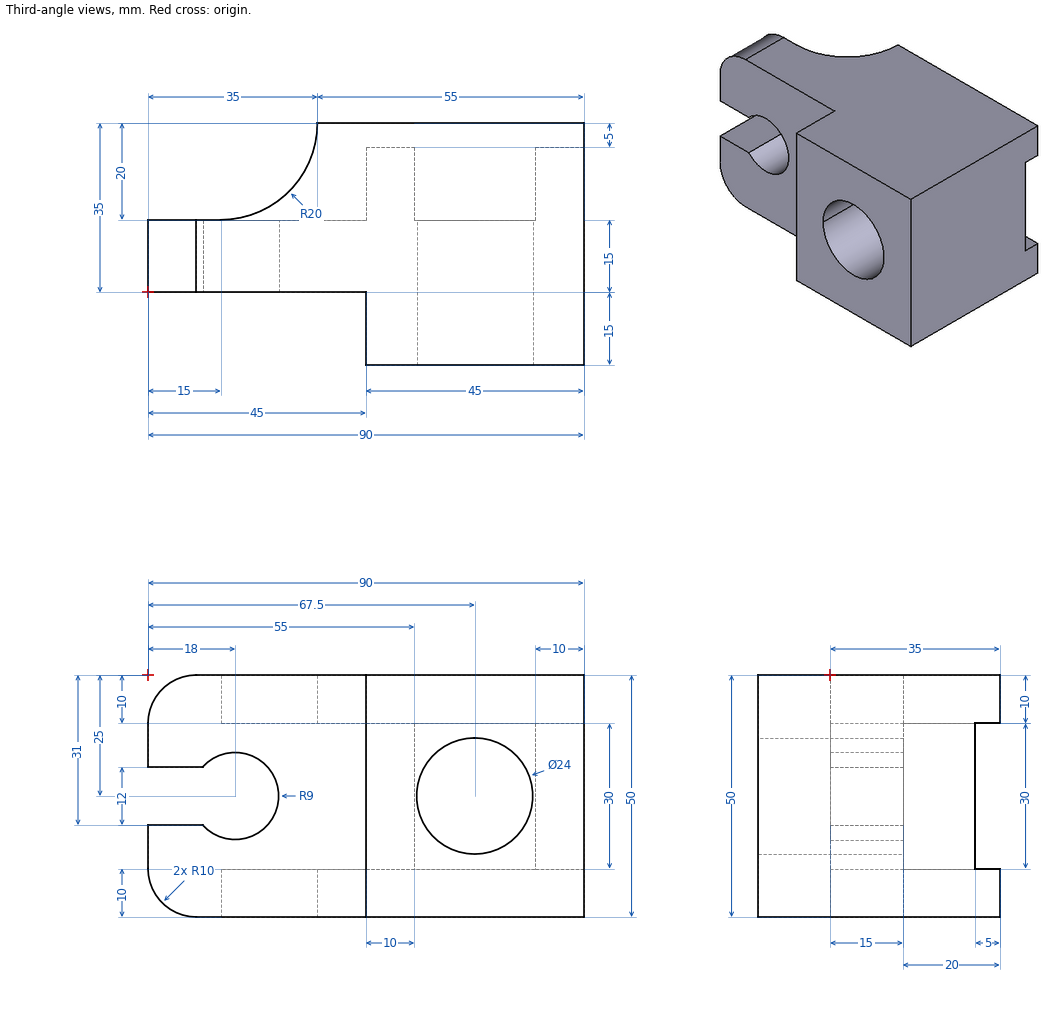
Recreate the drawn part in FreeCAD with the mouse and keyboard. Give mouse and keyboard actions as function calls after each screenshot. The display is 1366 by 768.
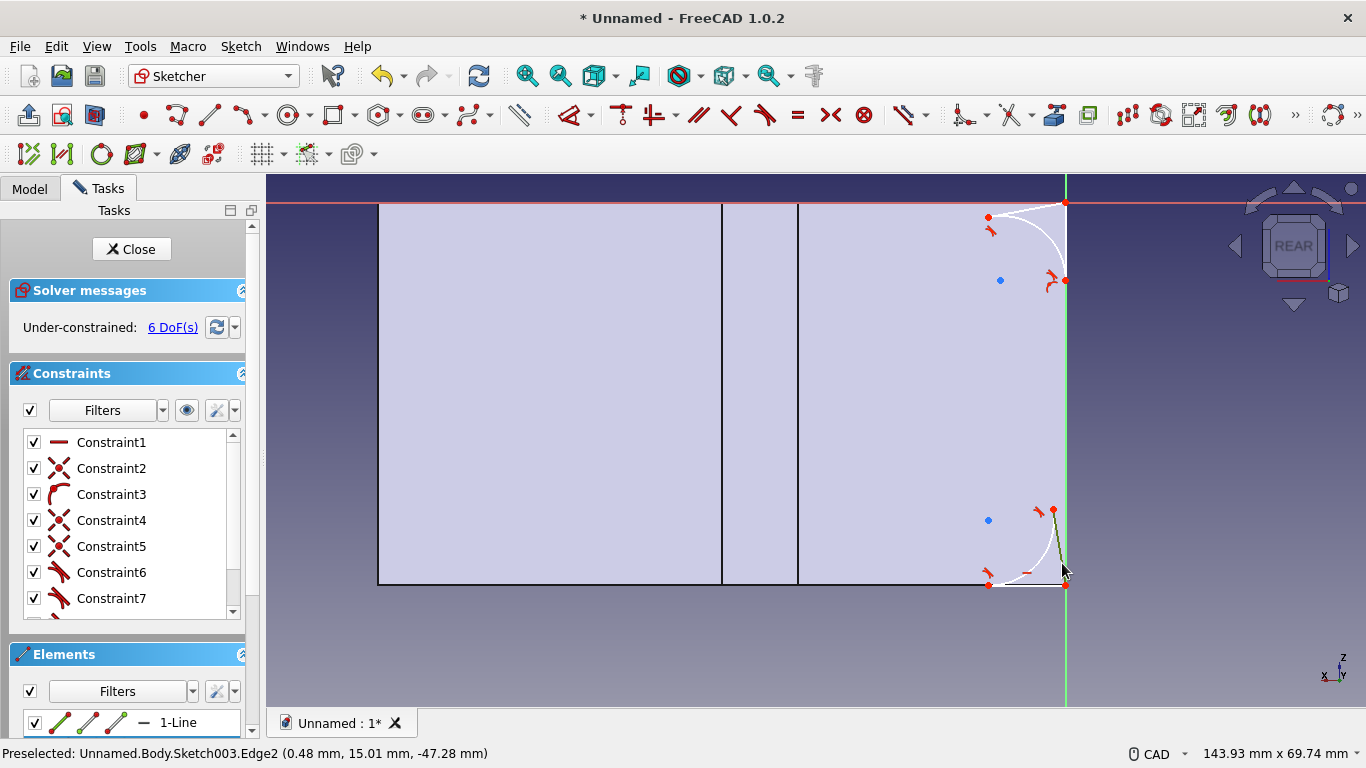
key(v)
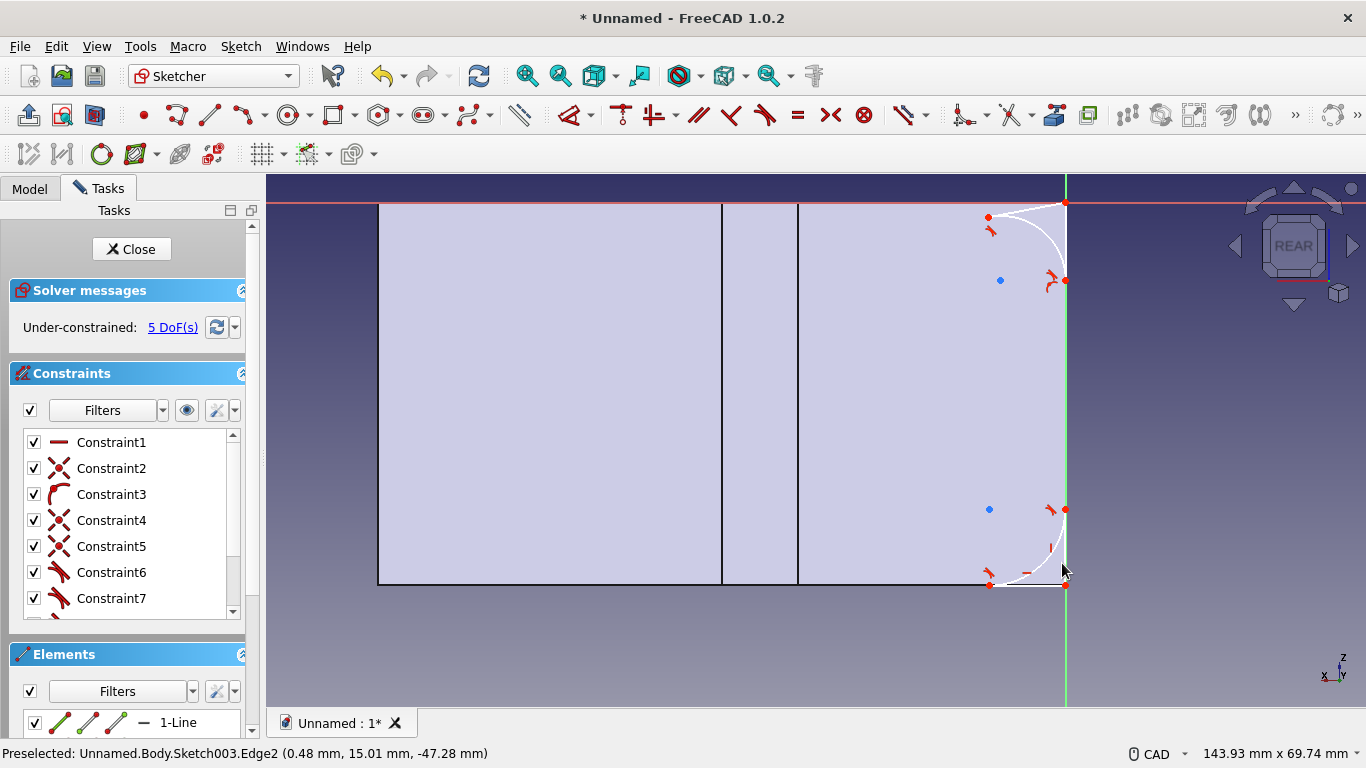
click(1050, 206)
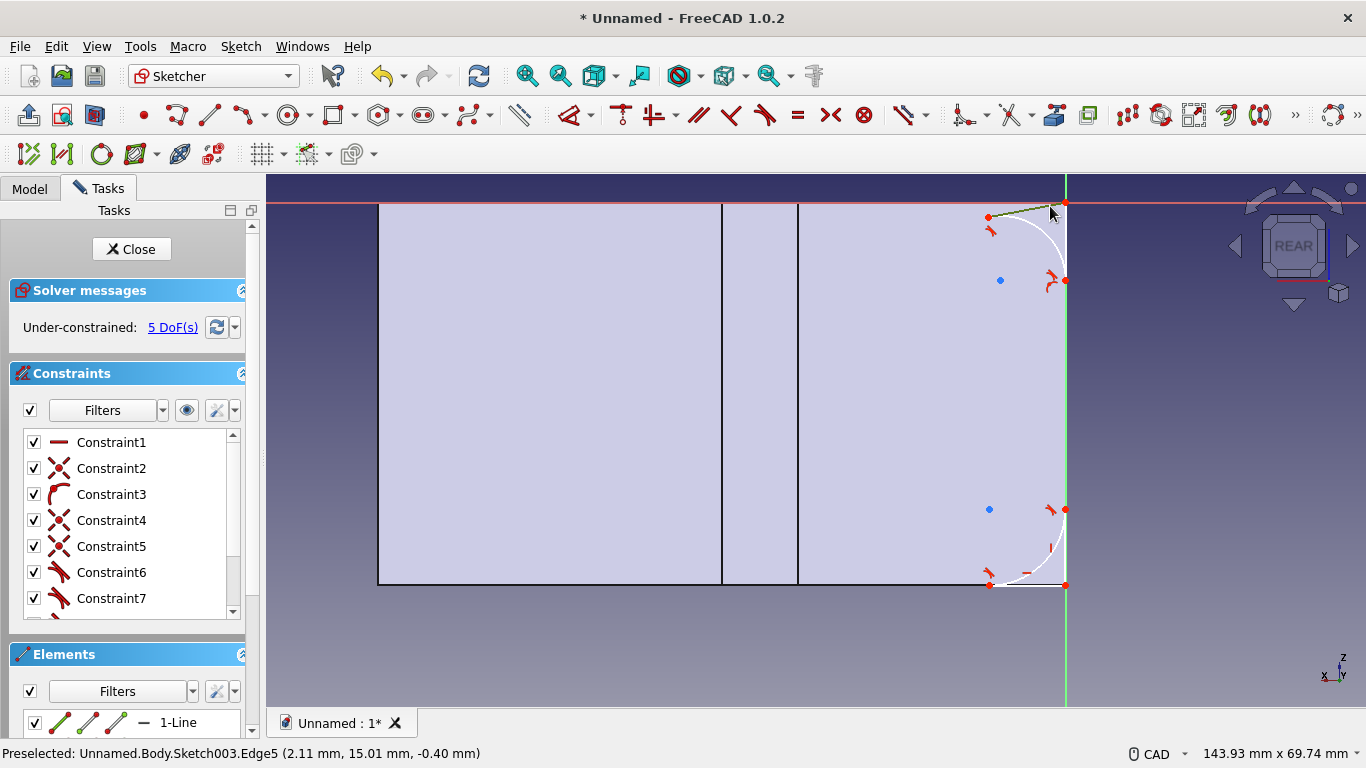
click(676, 116)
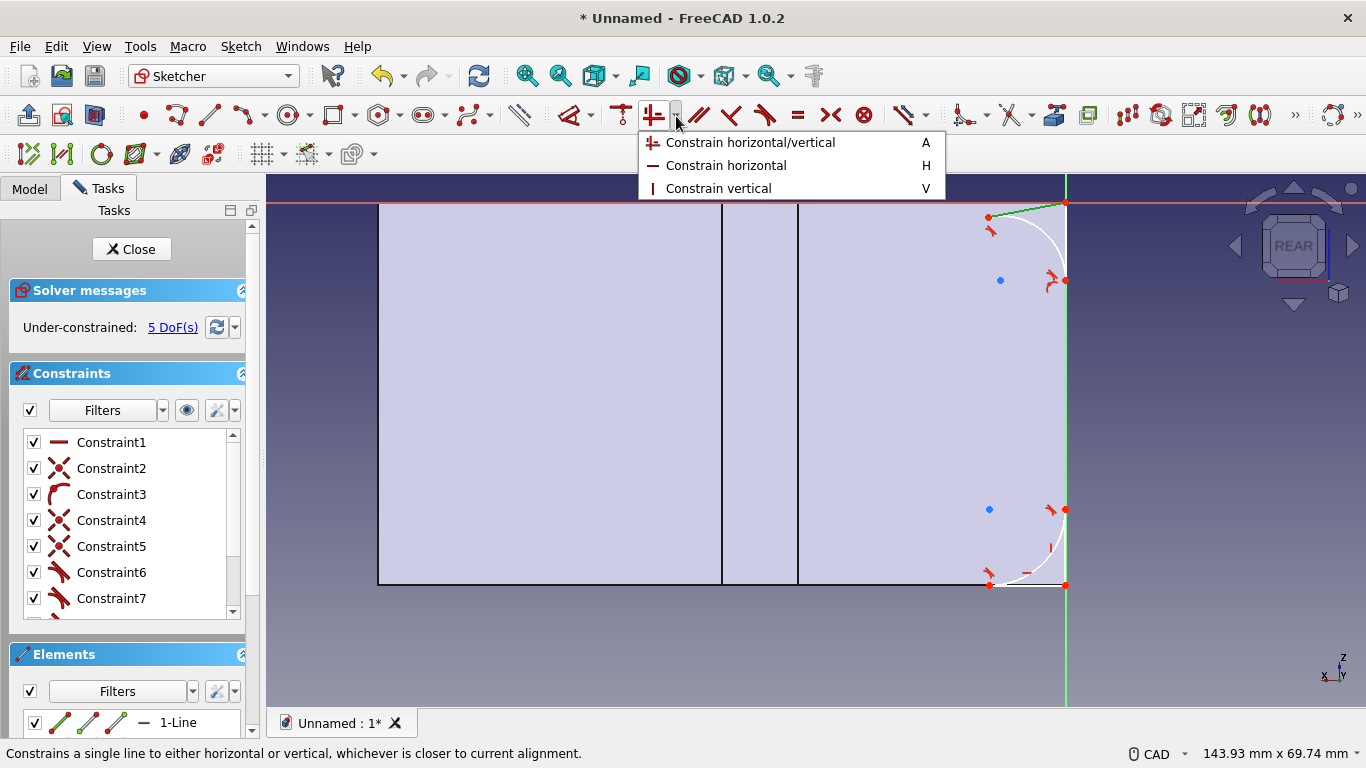
click(792, 166)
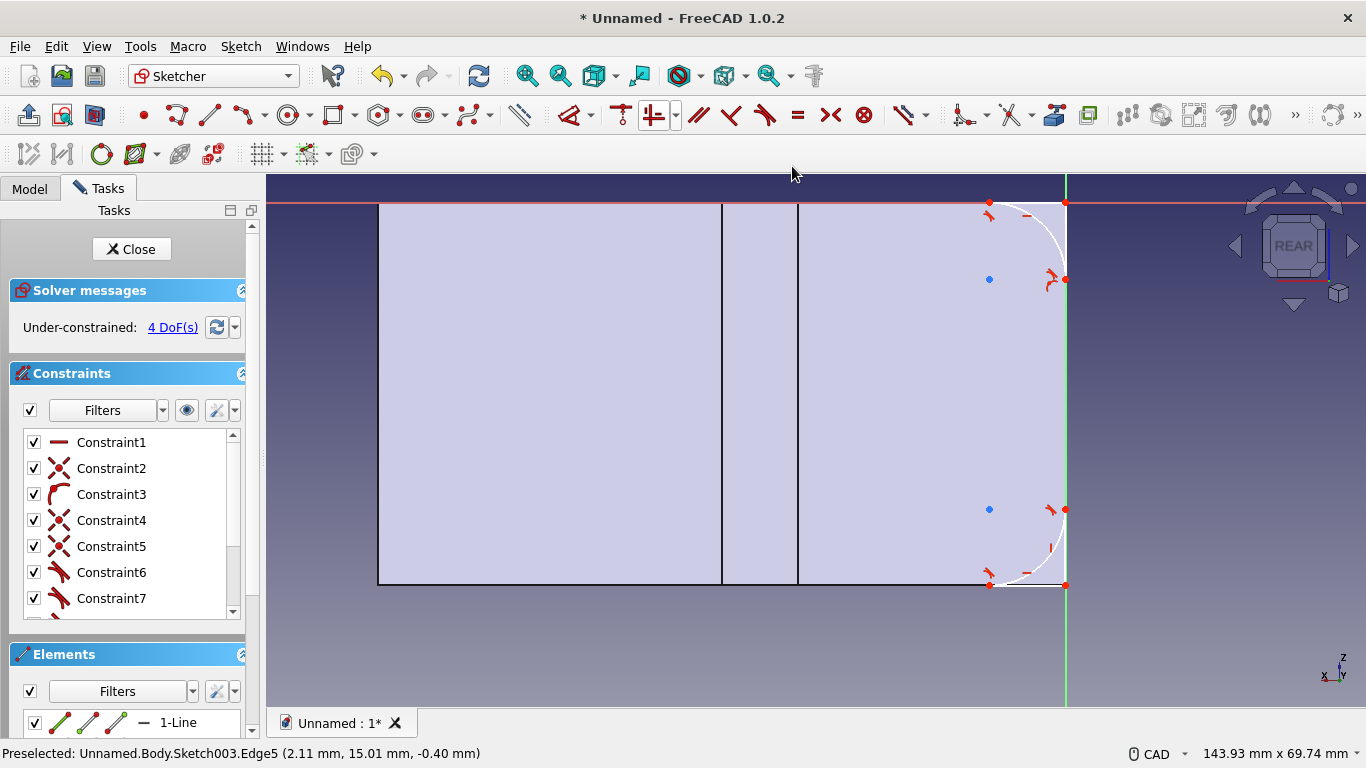
click(1043, 563)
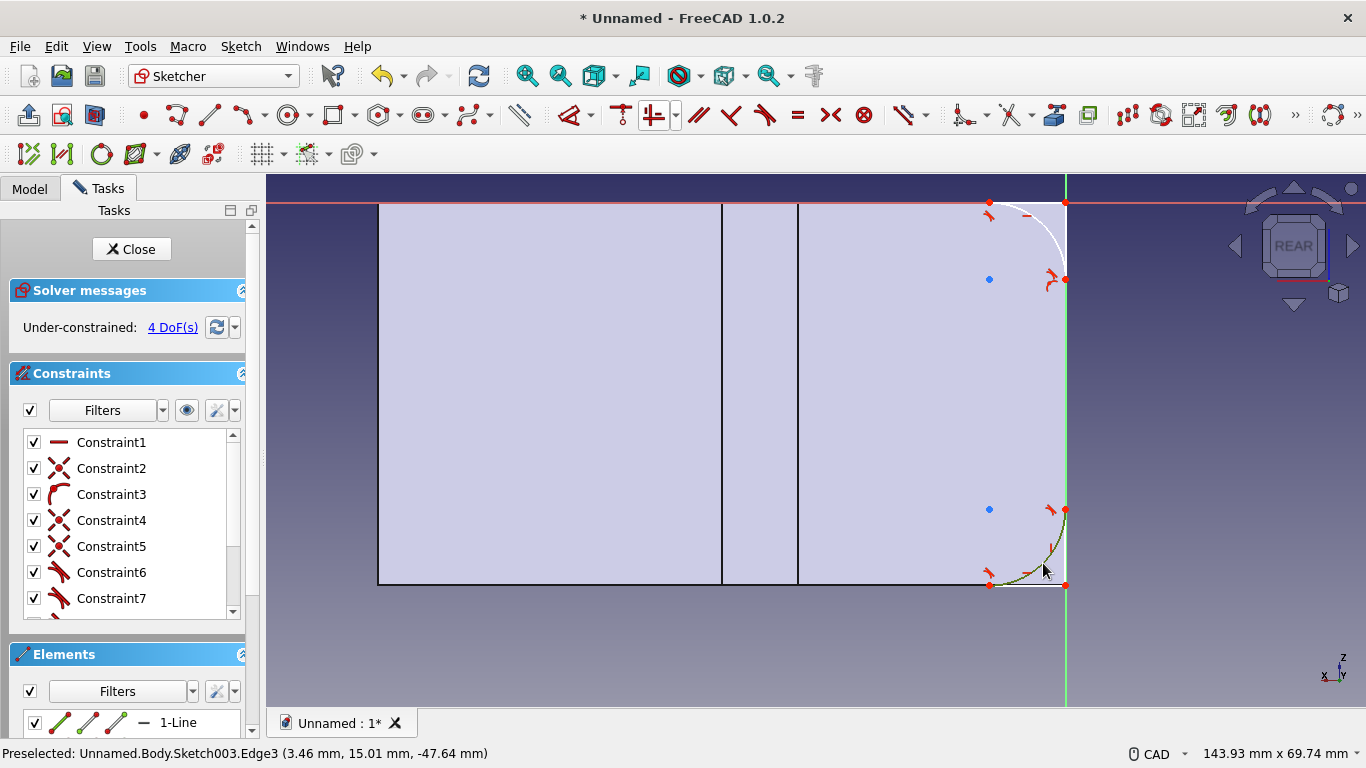
click(1043, 225)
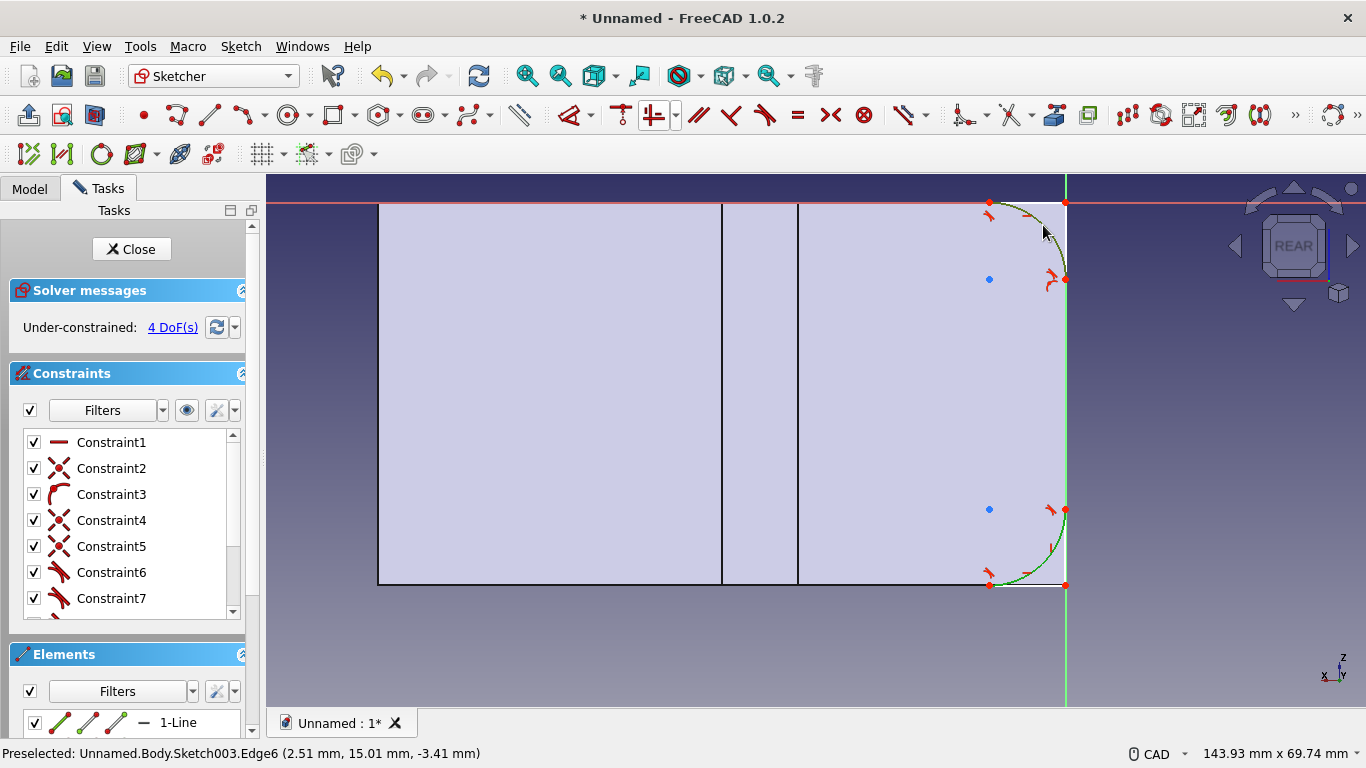
click(798, 116)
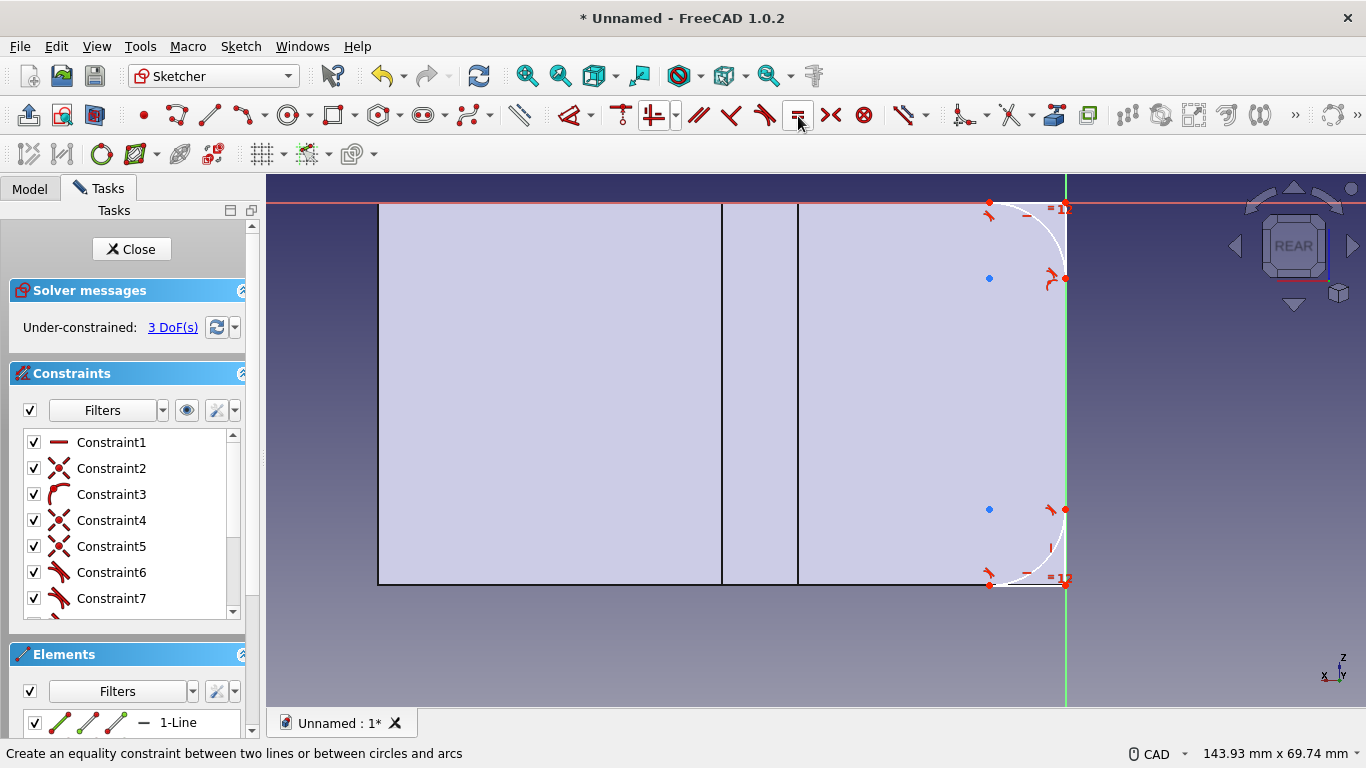
key(d)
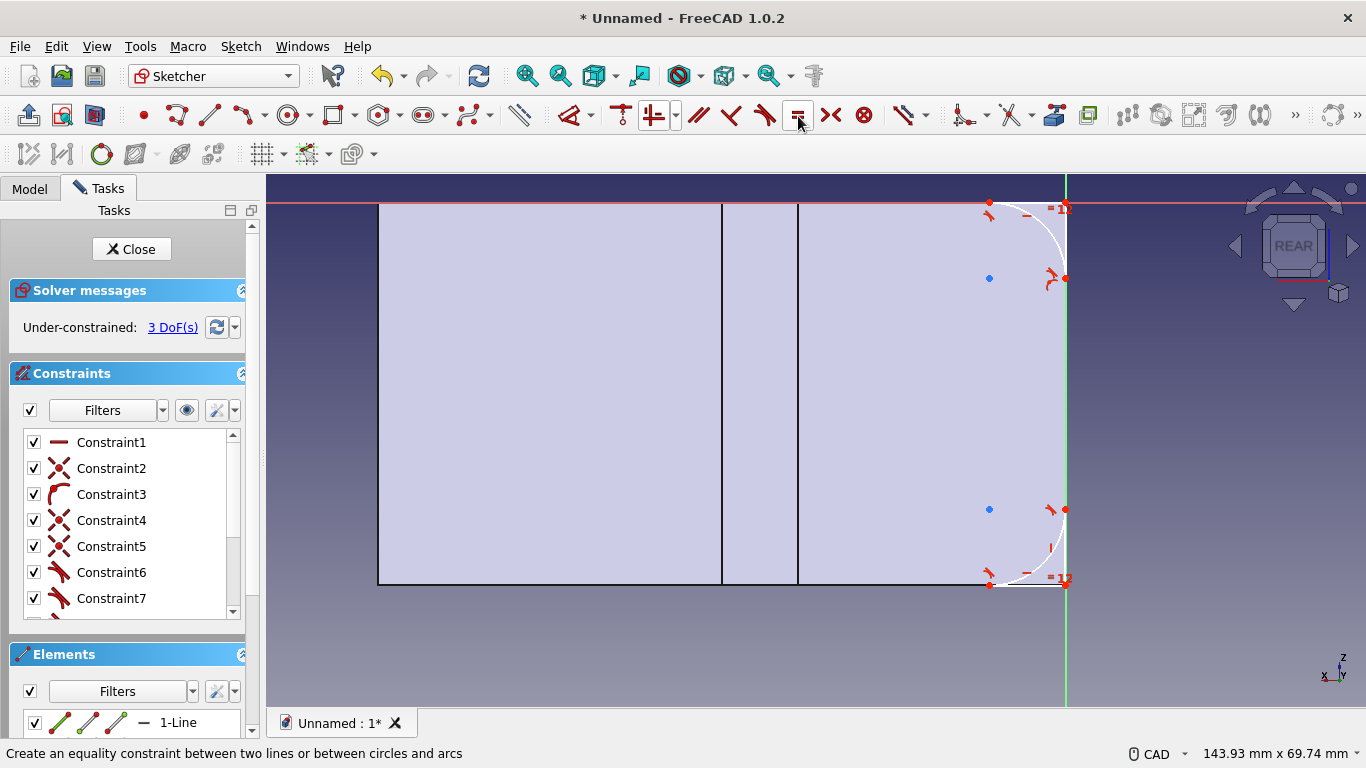
click(1043, 563)
click(1020, 613)